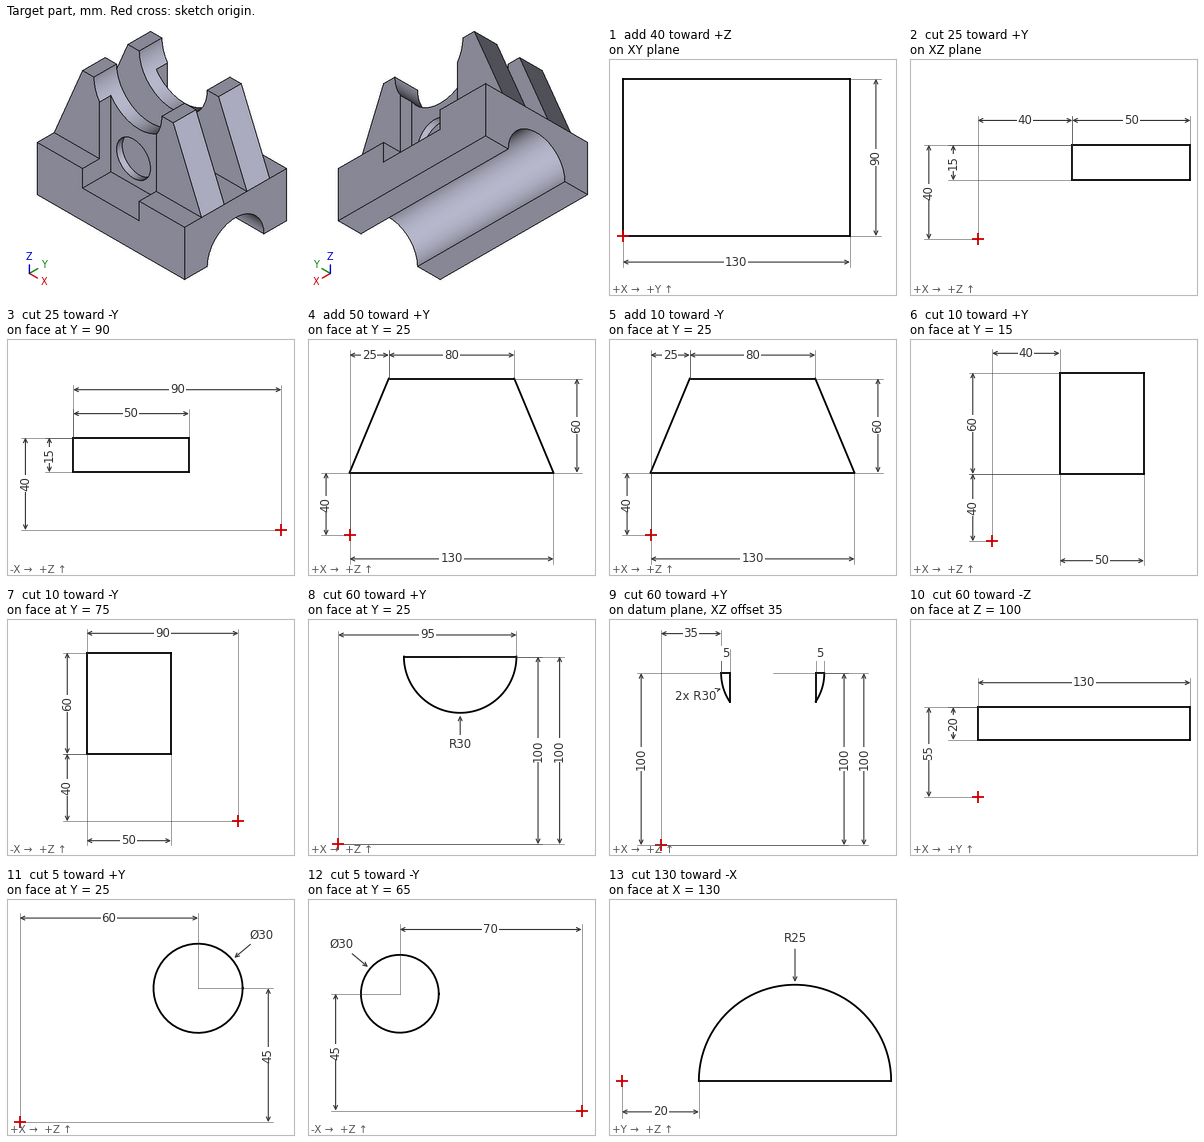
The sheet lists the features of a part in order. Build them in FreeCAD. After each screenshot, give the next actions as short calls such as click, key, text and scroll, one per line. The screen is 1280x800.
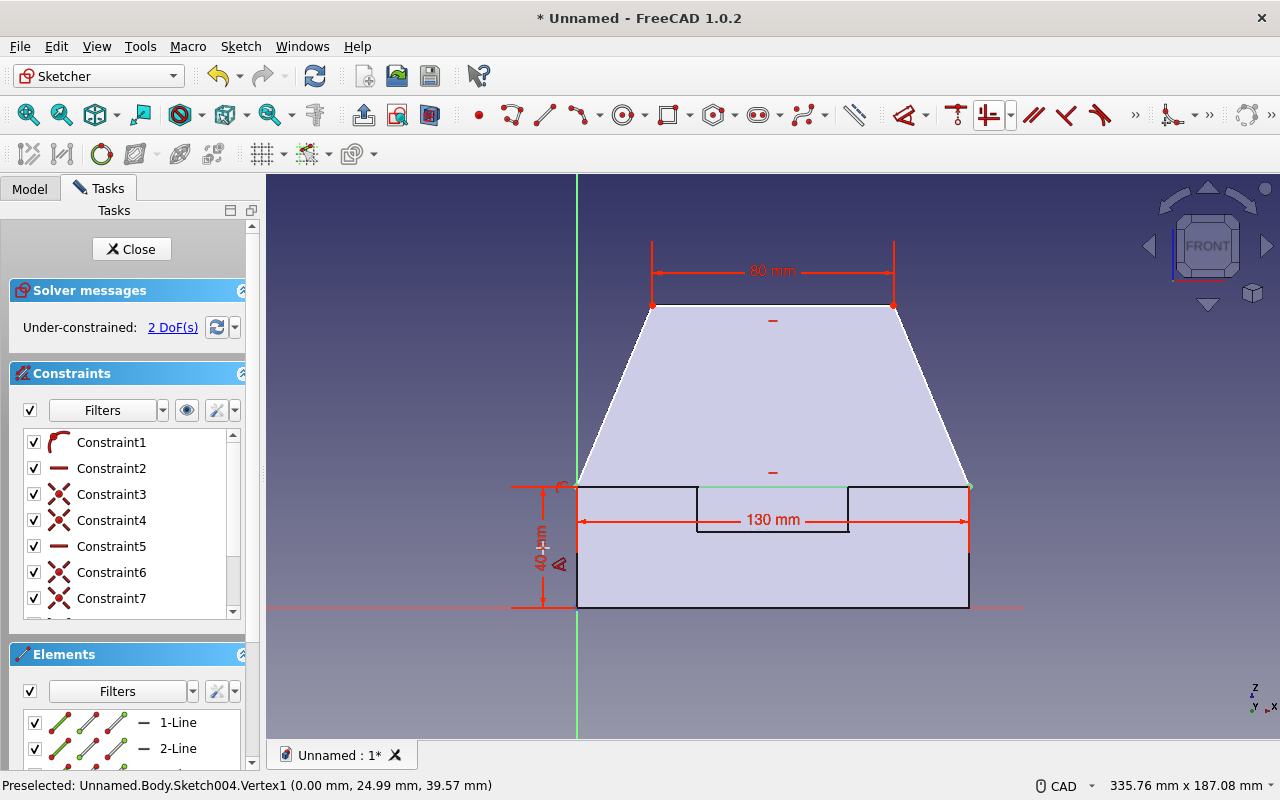
click(652, 306)
click(614, 642)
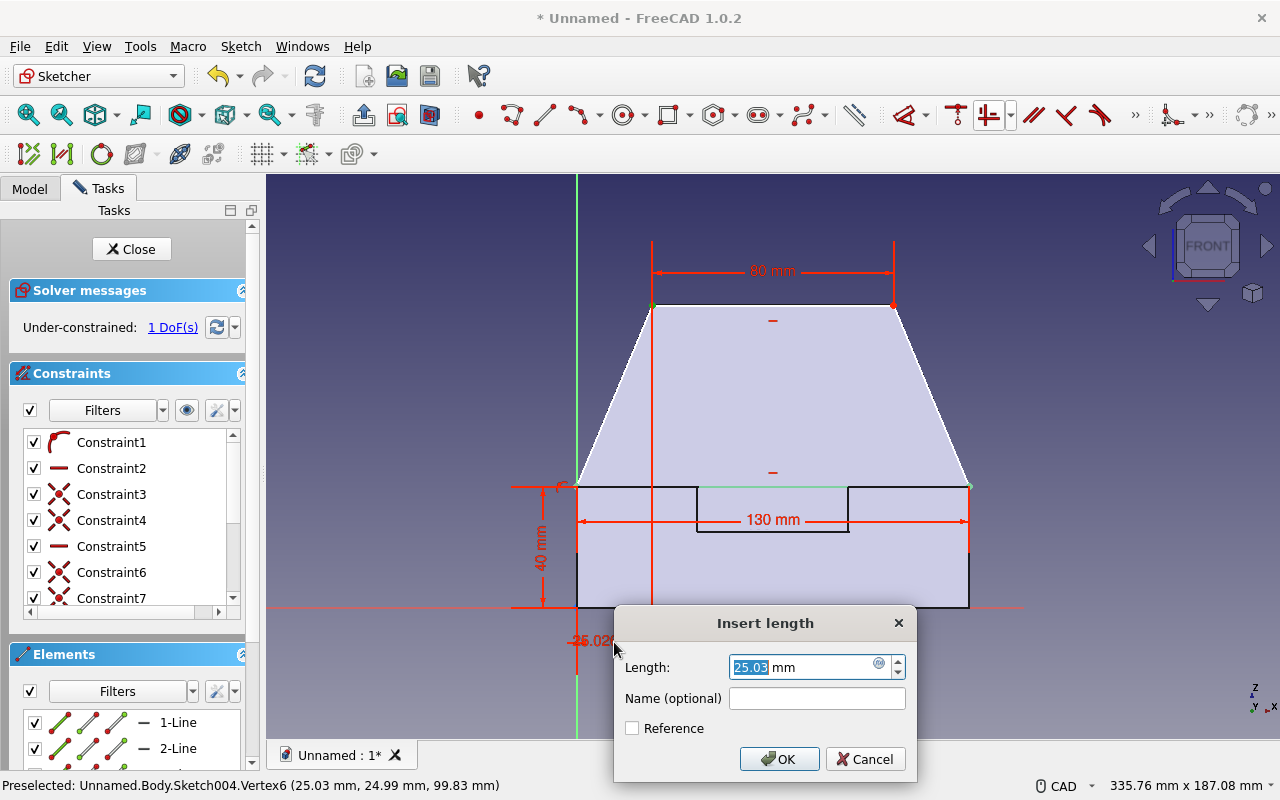
text(25)
key(Return)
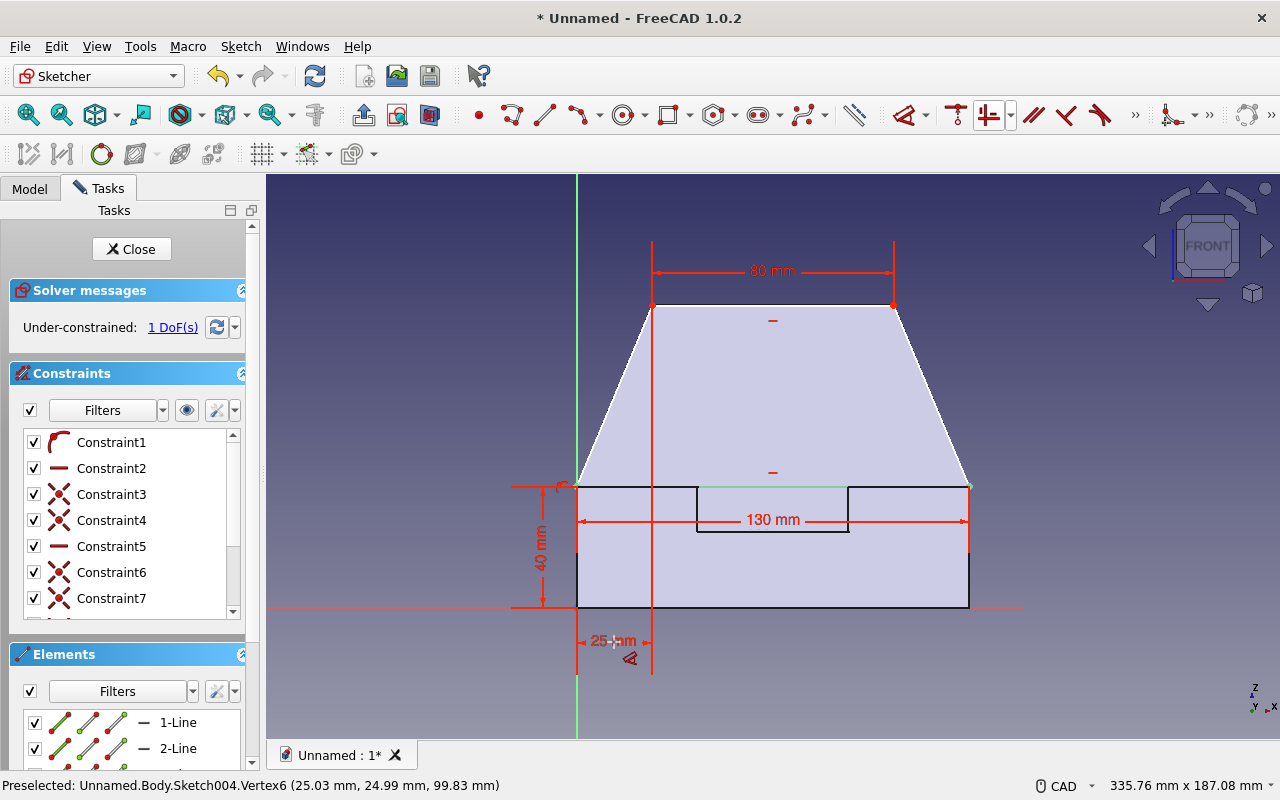
click(947, 432)
click(1003, 396)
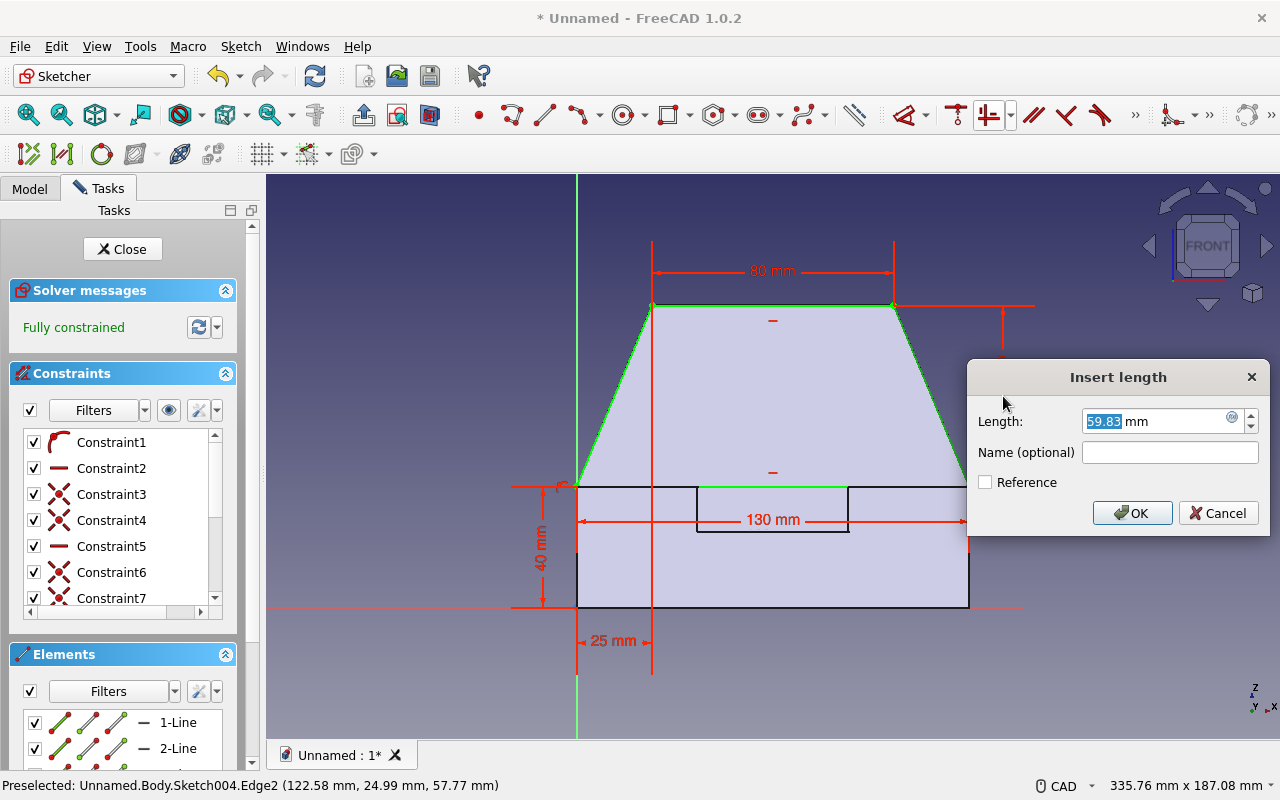
text(60)
key(Return)
key(Escape)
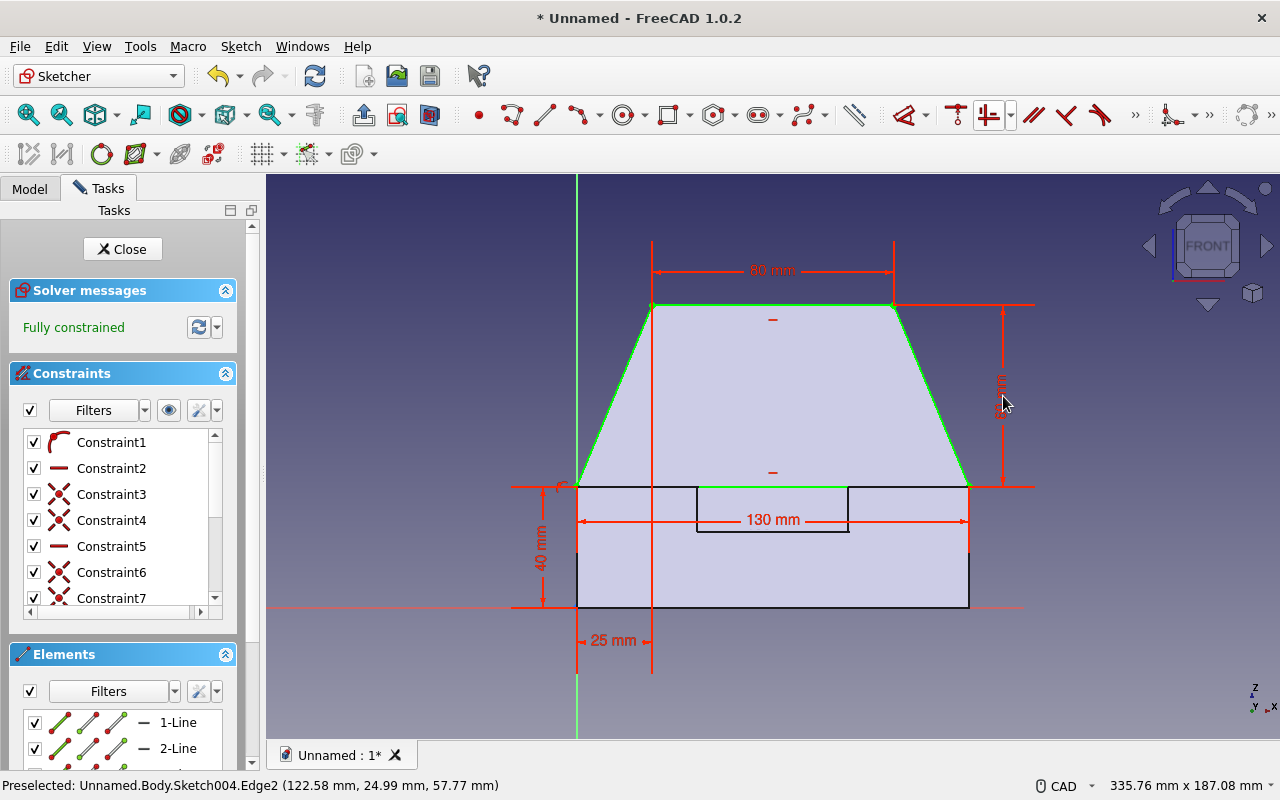
click(123, 249)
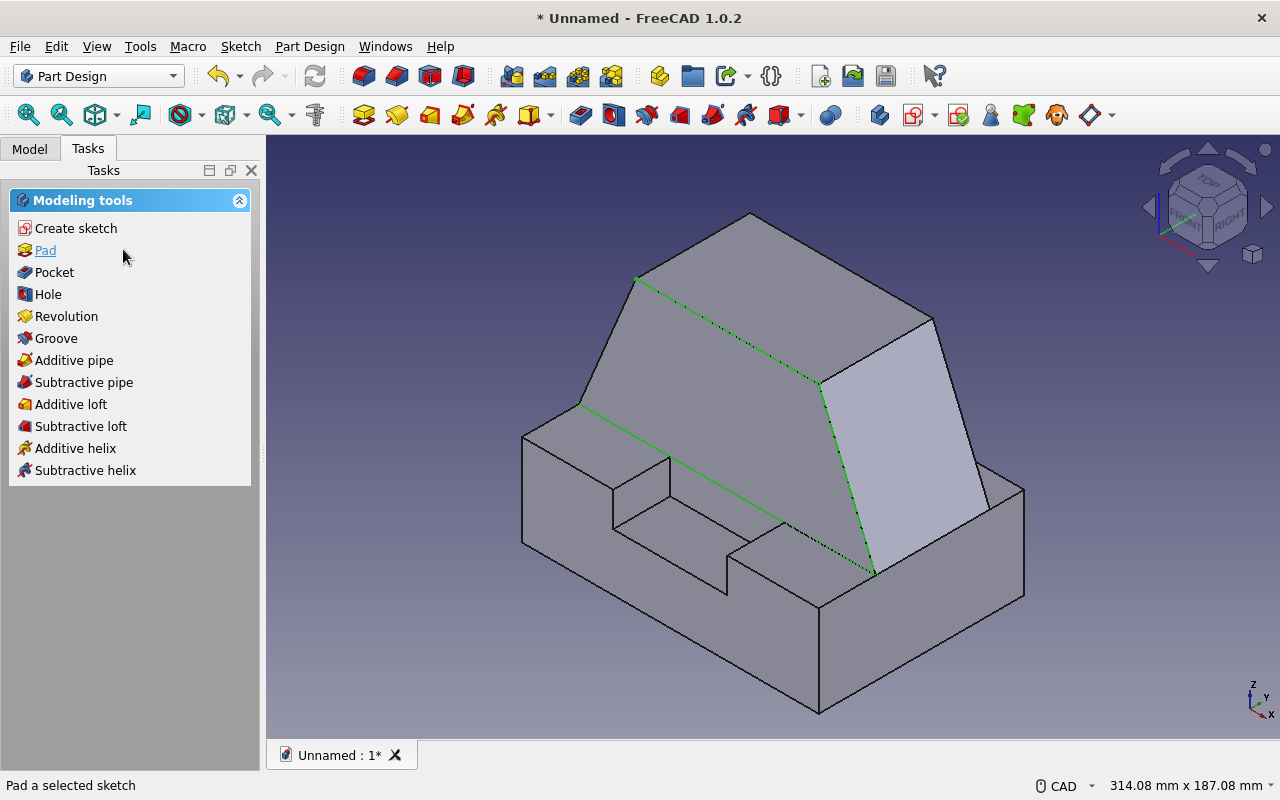
click(364, 116)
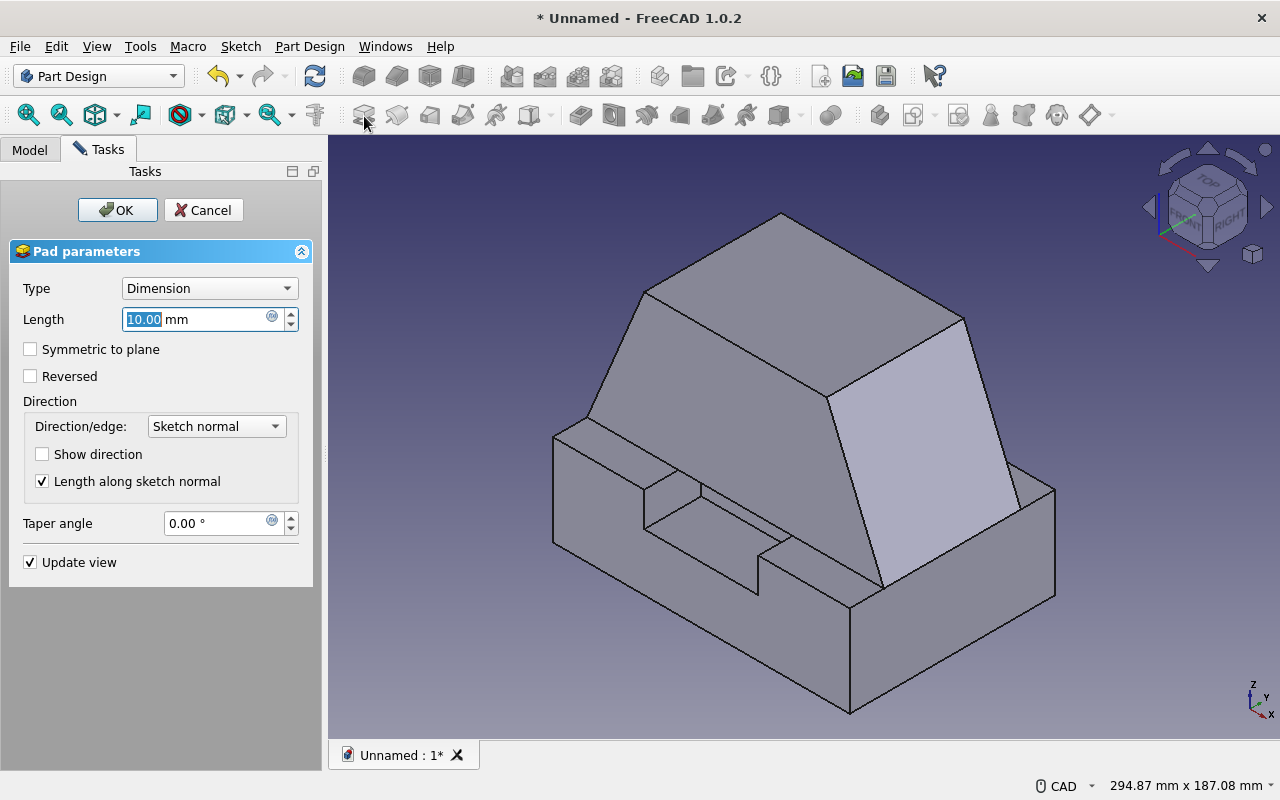
text(10)
key(Tab)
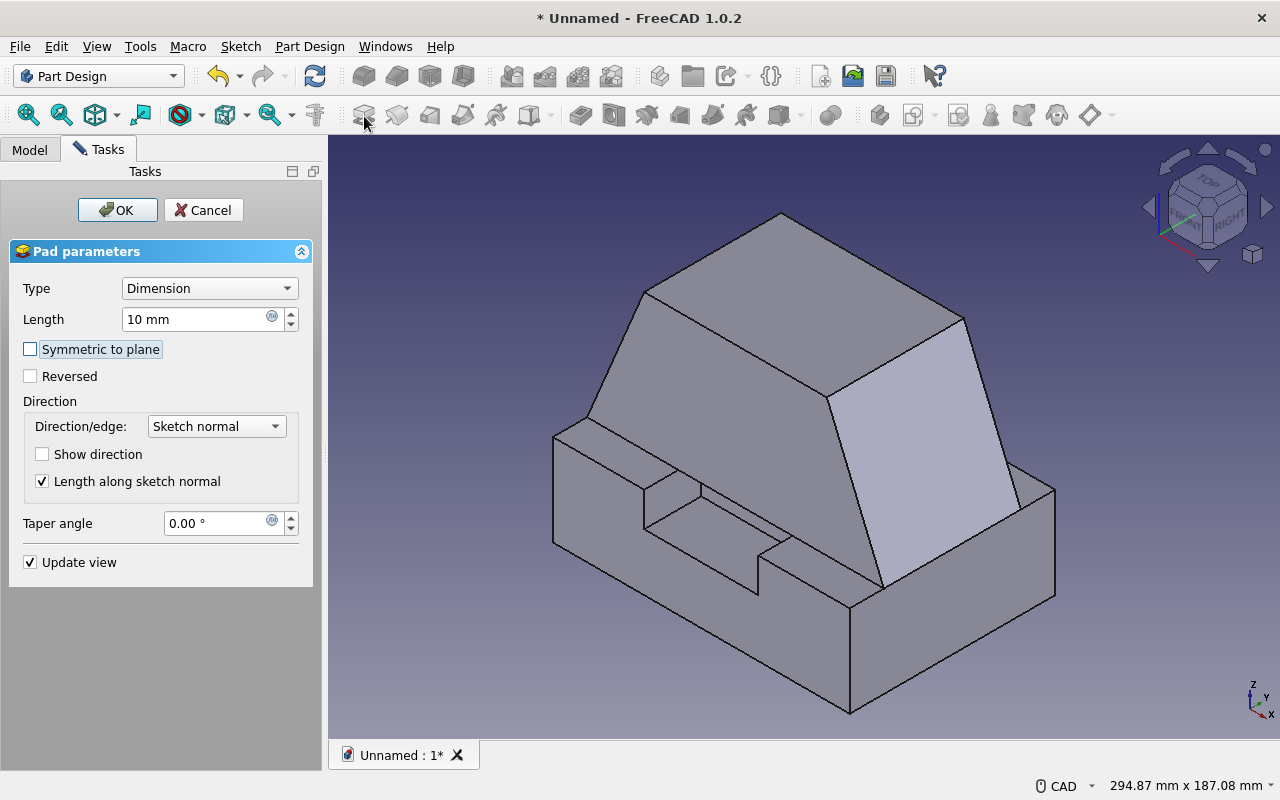
click(118, 210)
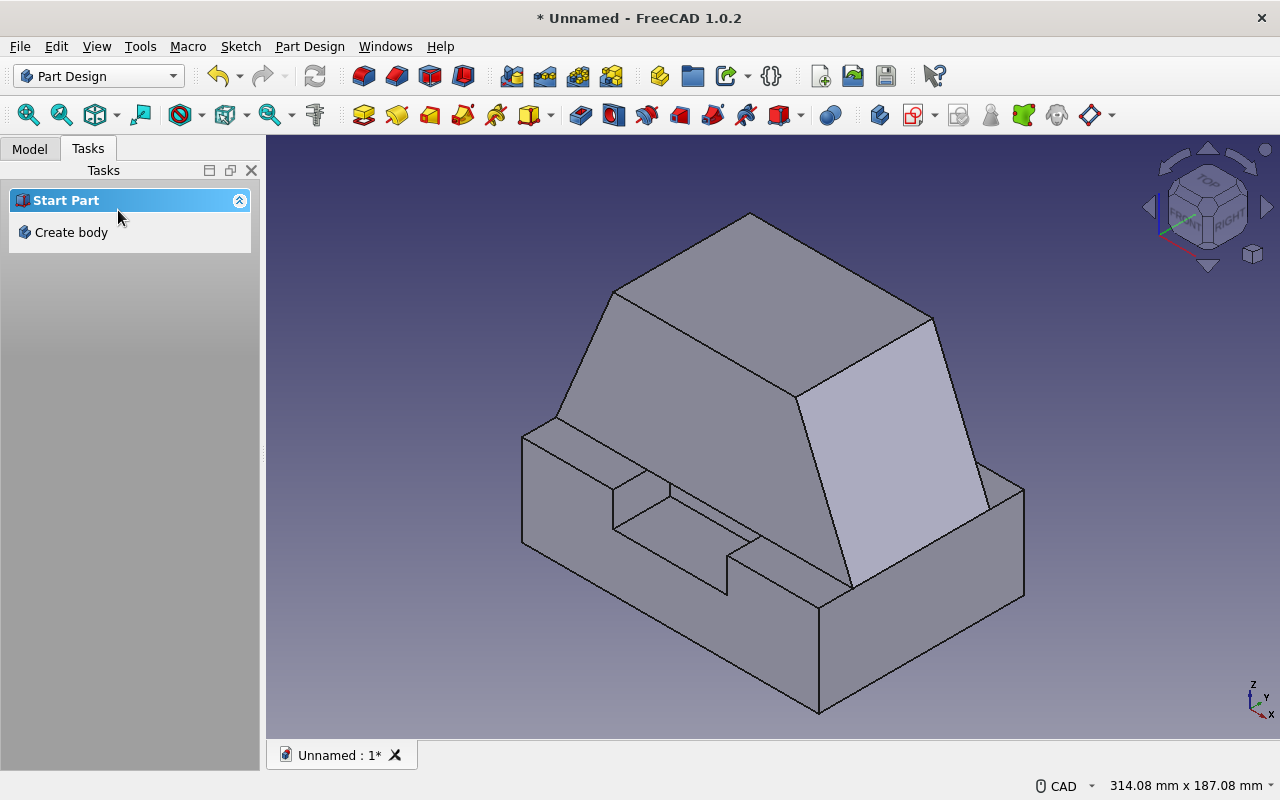
click(747, 447)